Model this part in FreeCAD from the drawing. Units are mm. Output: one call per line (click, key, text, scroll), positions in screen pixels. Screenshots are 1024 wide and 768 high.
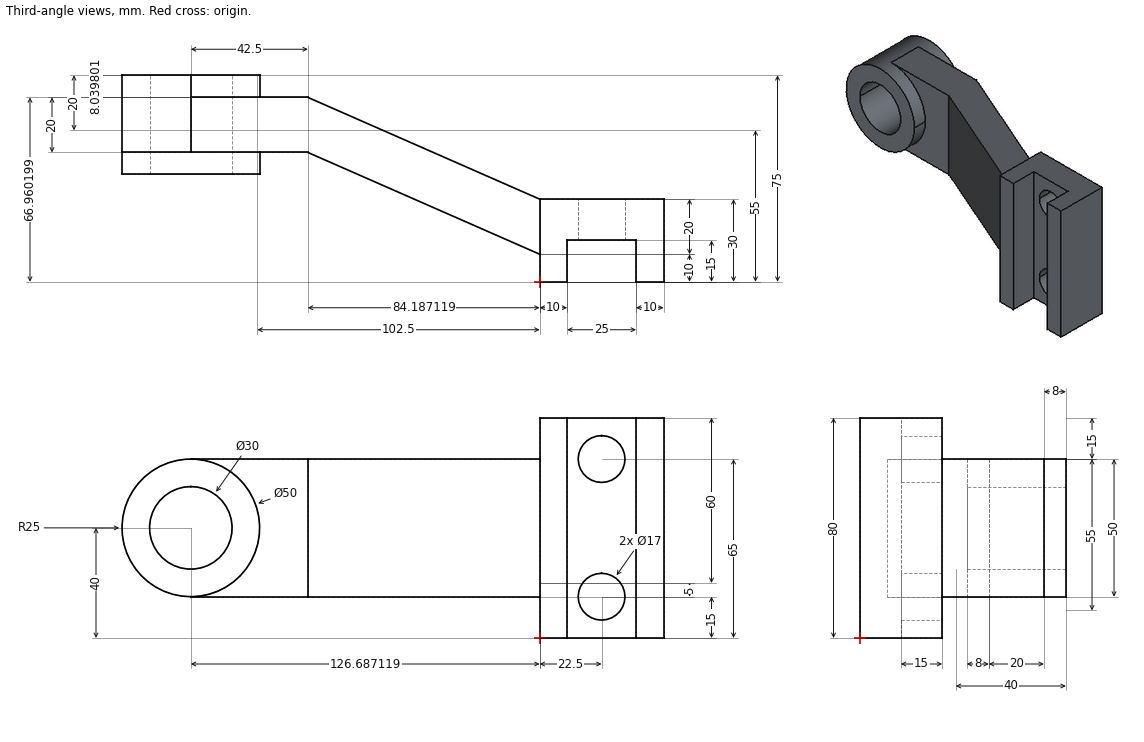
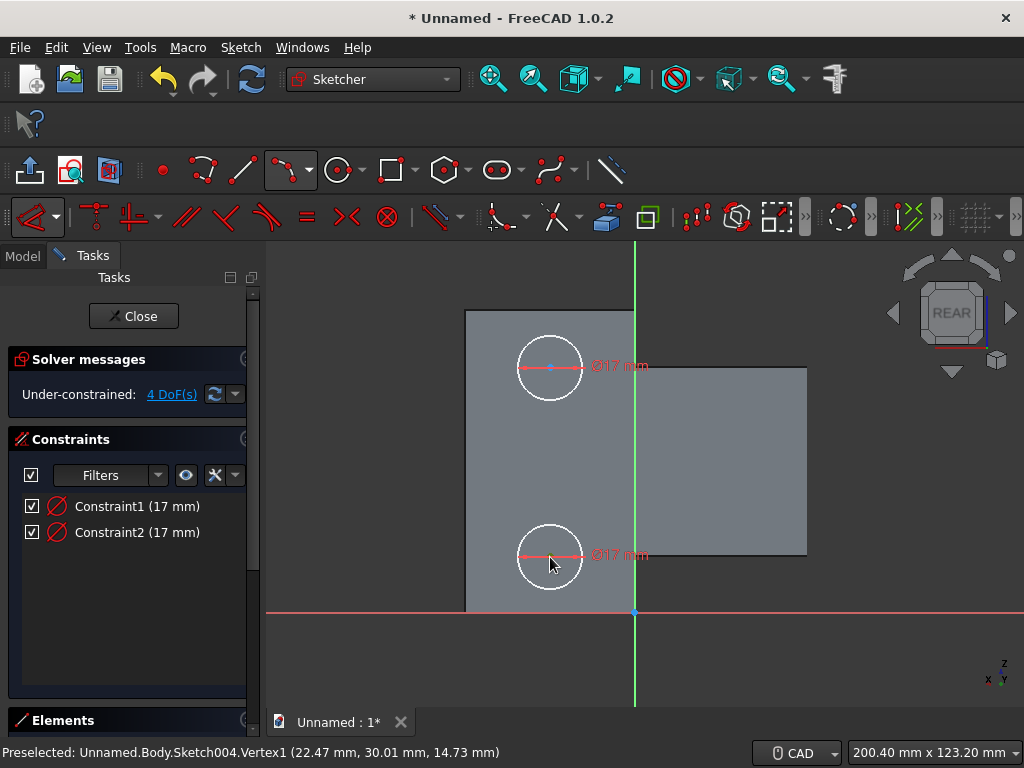
click(550, 368)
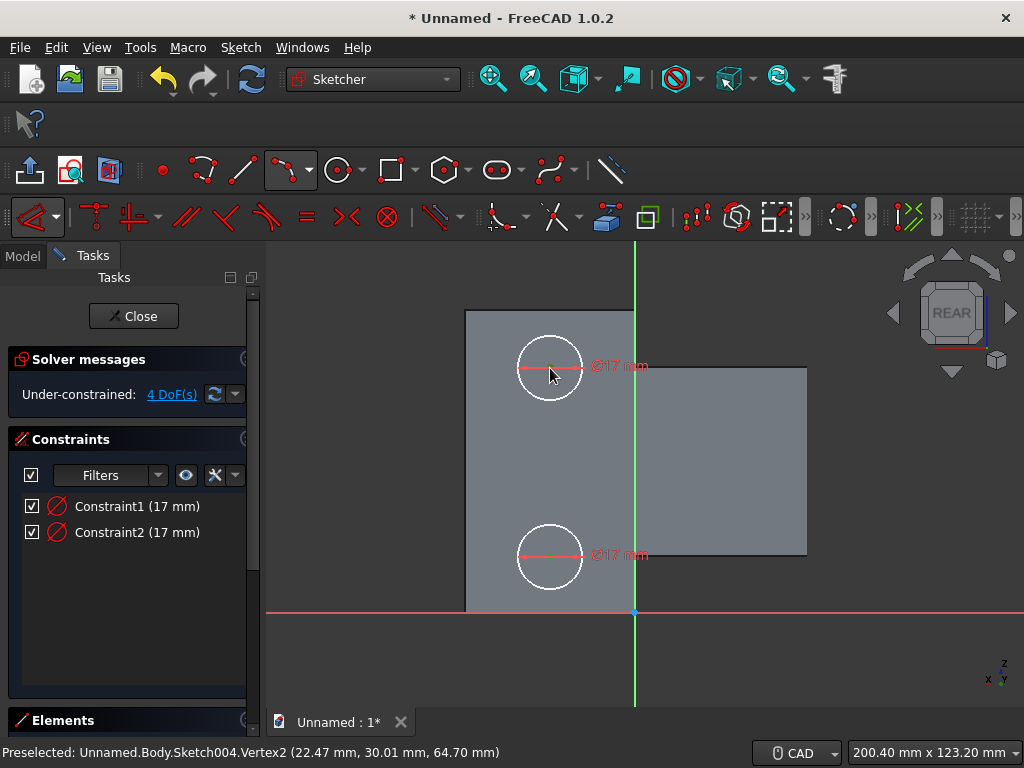
key(v)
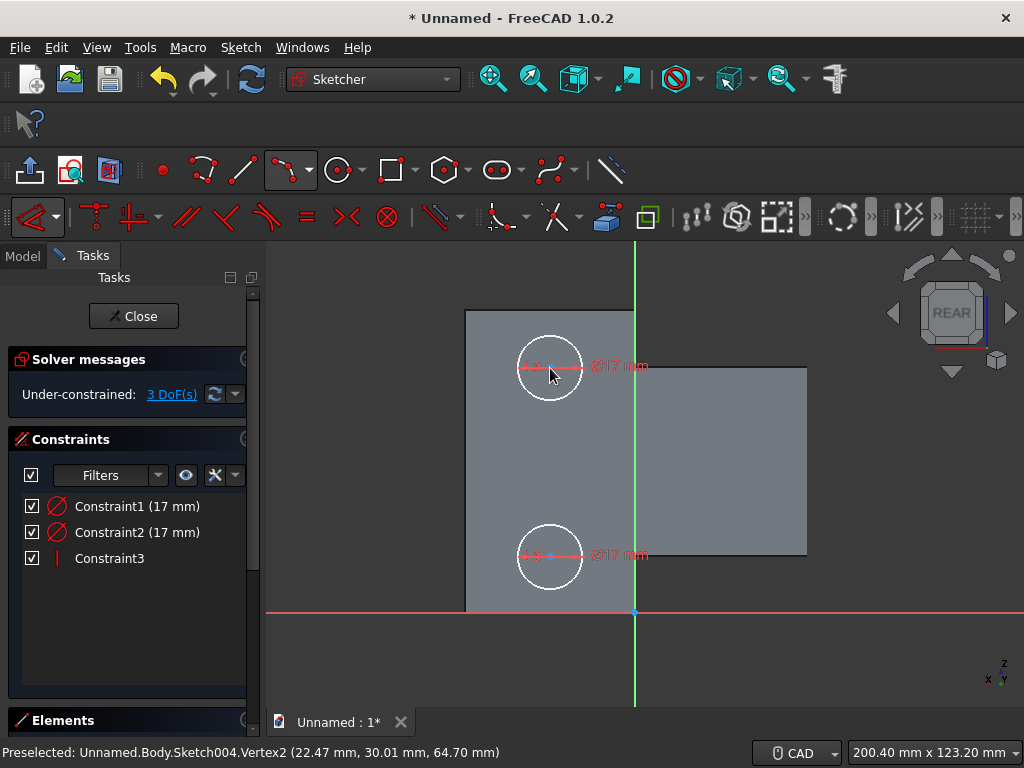
click(550, 557)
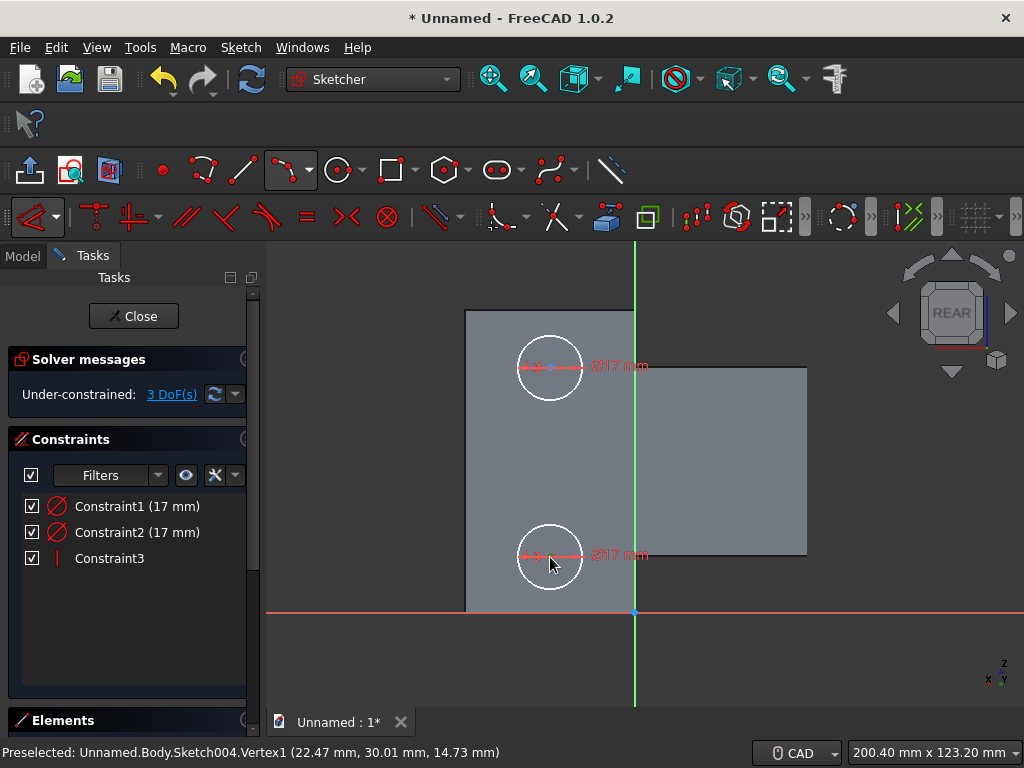
key(i)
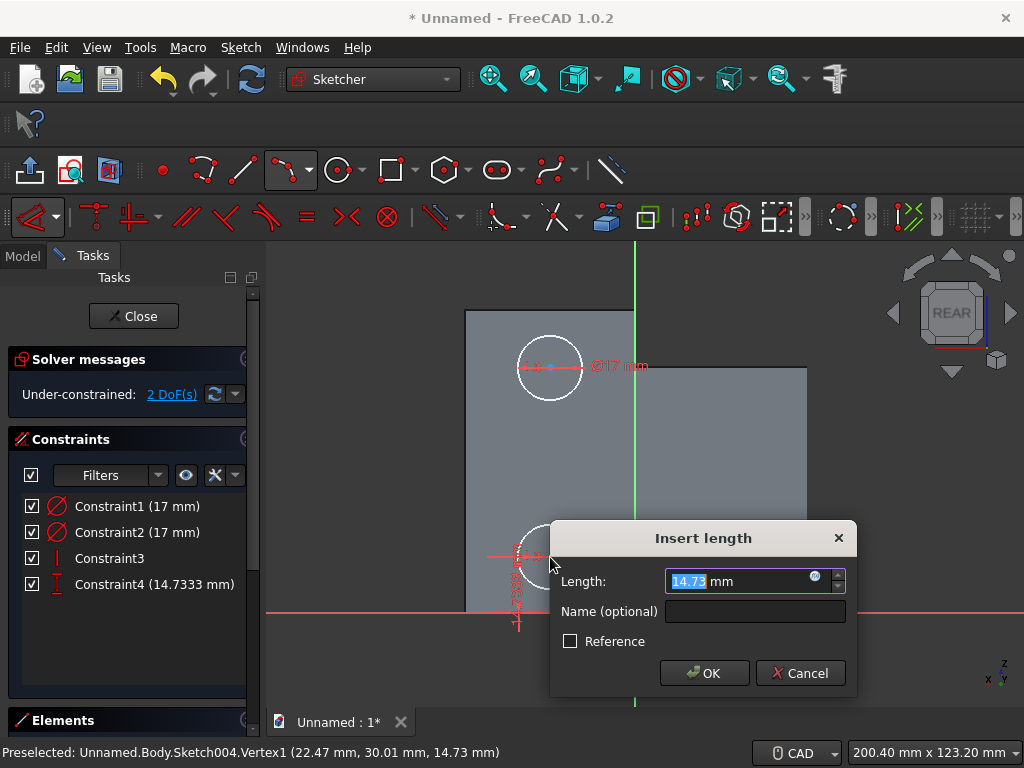
text(15)
key(Return)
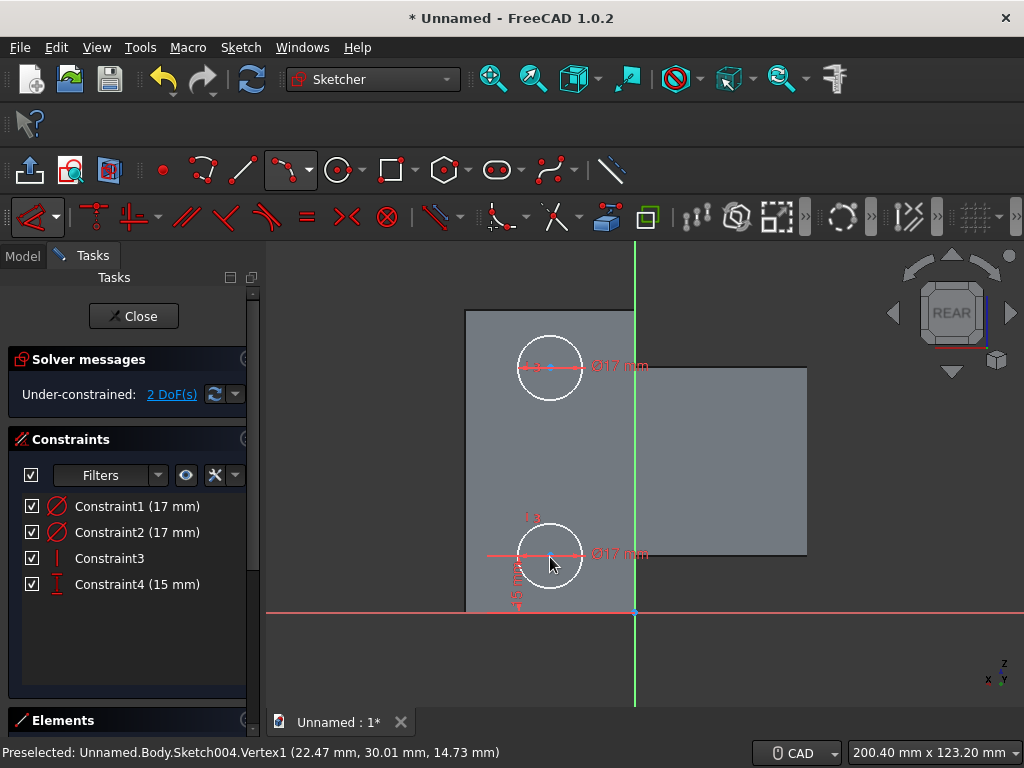
click(550, 368)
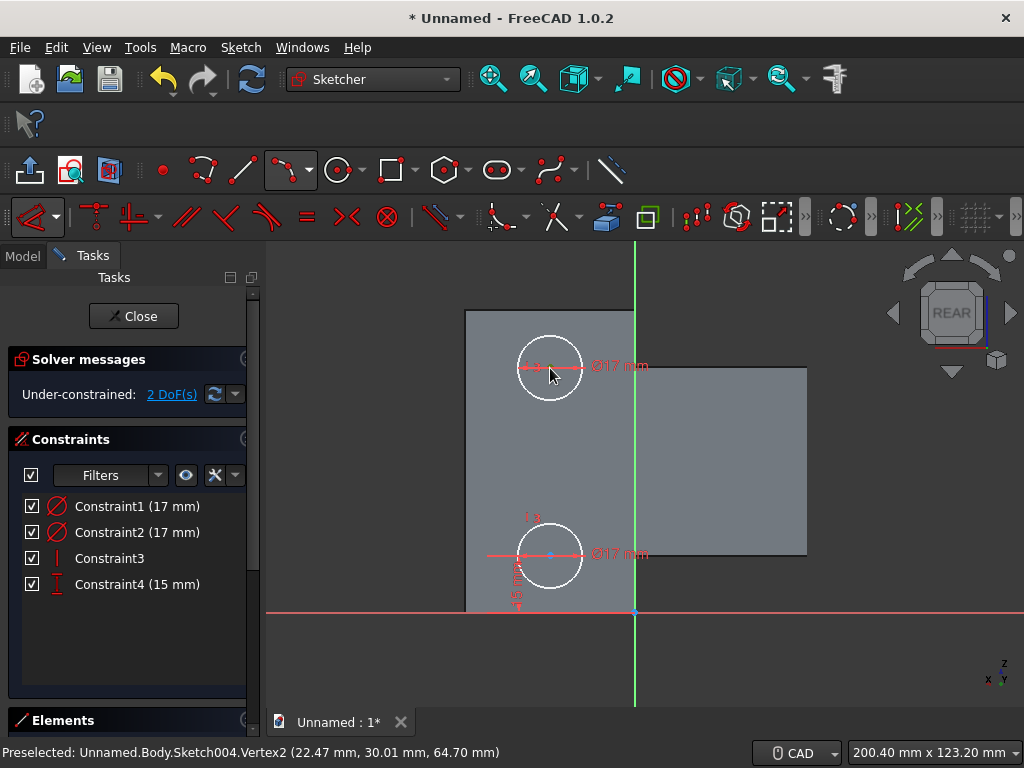
key(i)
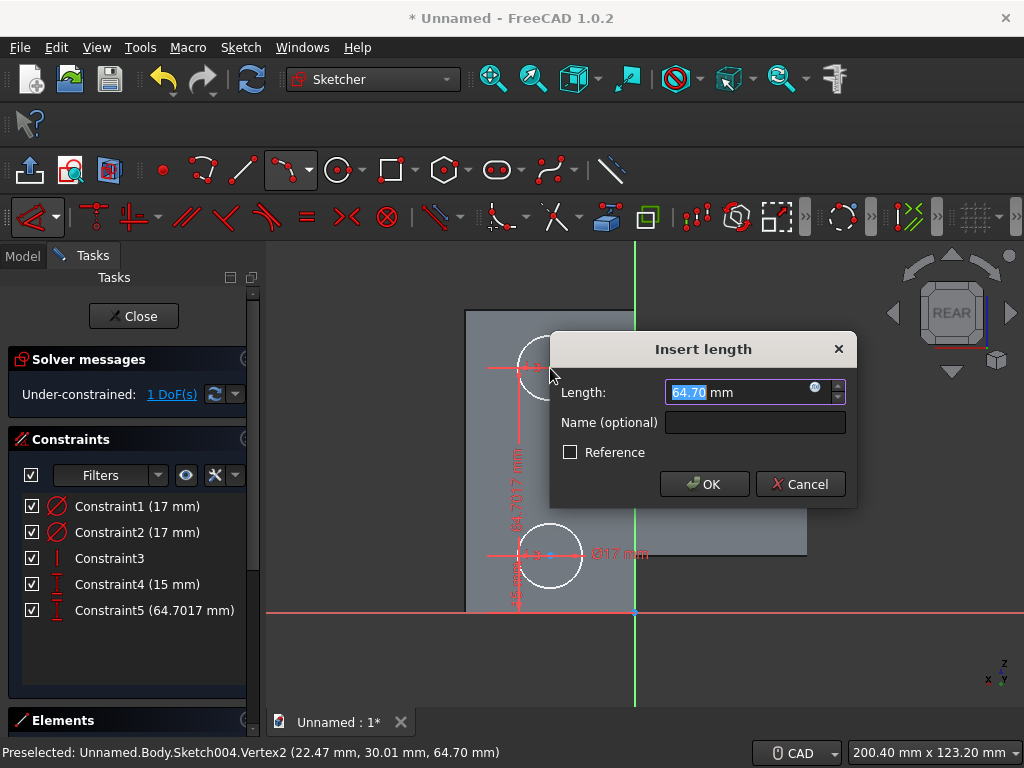
text(65)
key(Return)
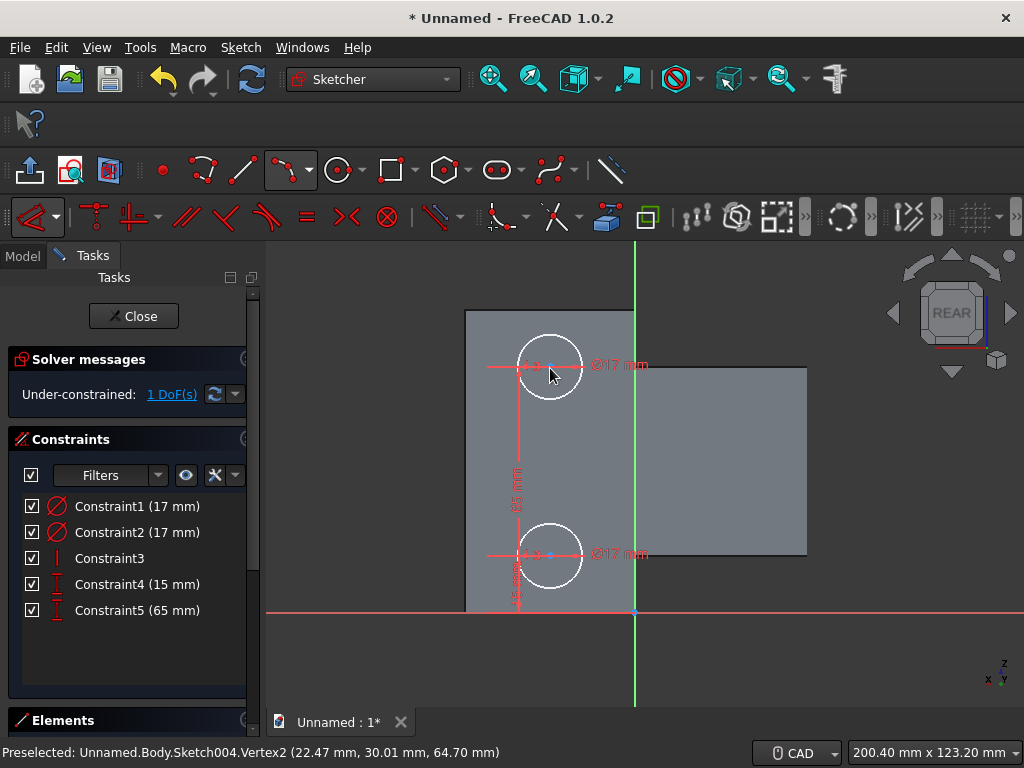
click(550, 556)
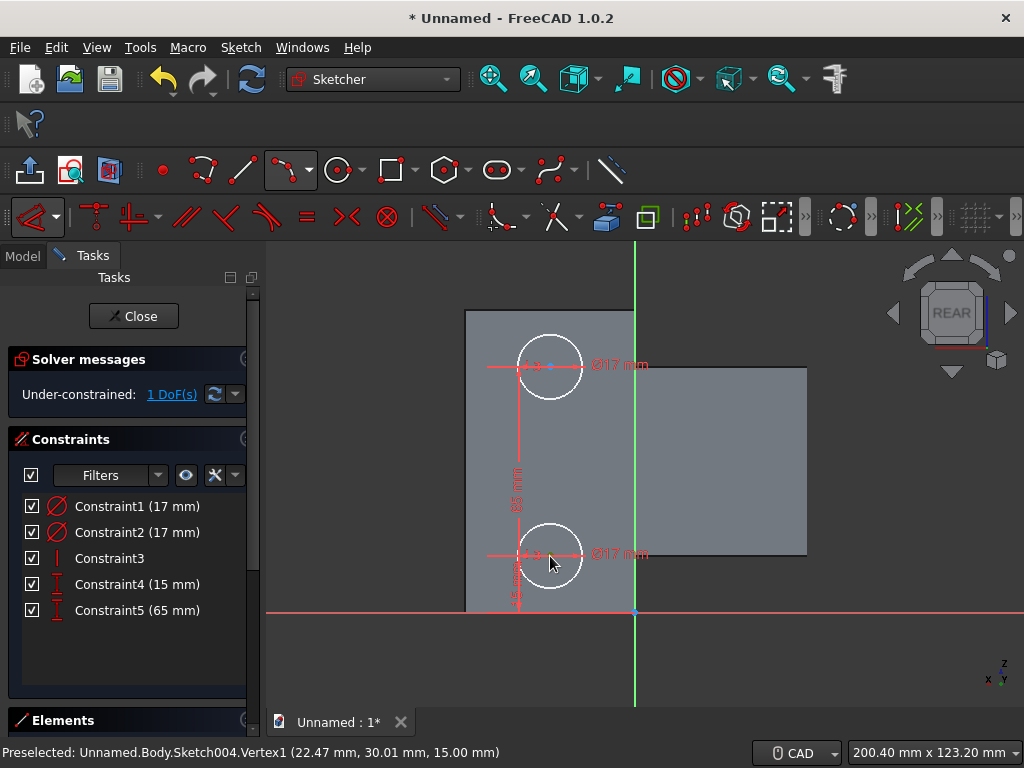
key(l)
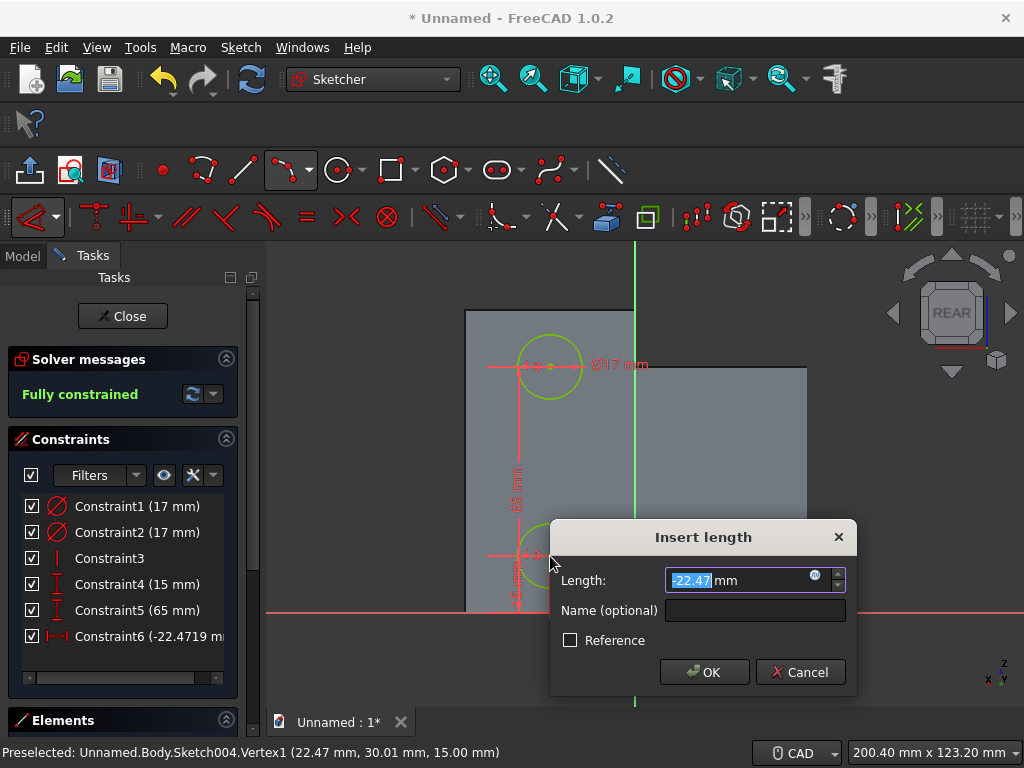
text(-22.5)
key(Return)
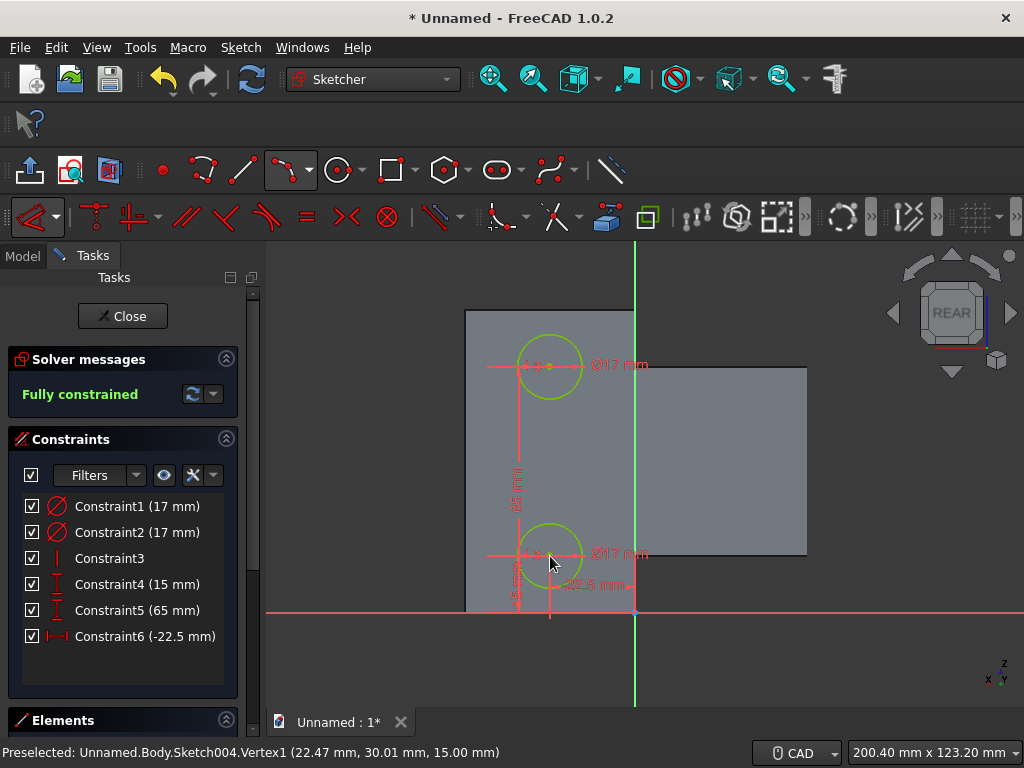
click(123, 316)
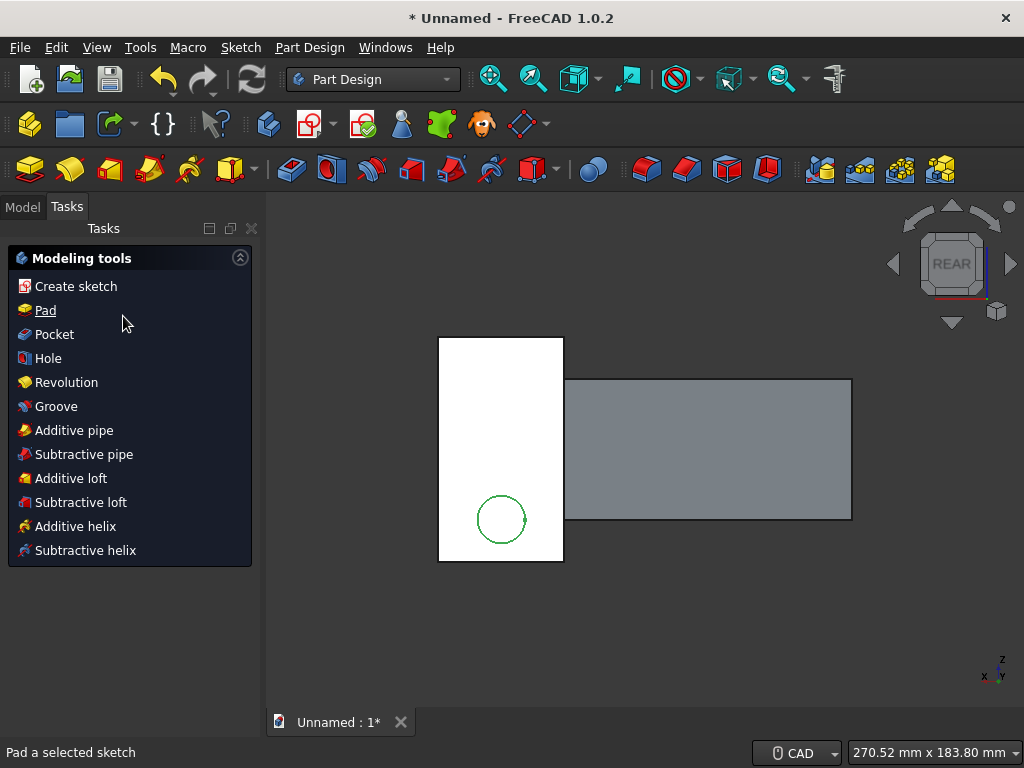
click(292, 170)